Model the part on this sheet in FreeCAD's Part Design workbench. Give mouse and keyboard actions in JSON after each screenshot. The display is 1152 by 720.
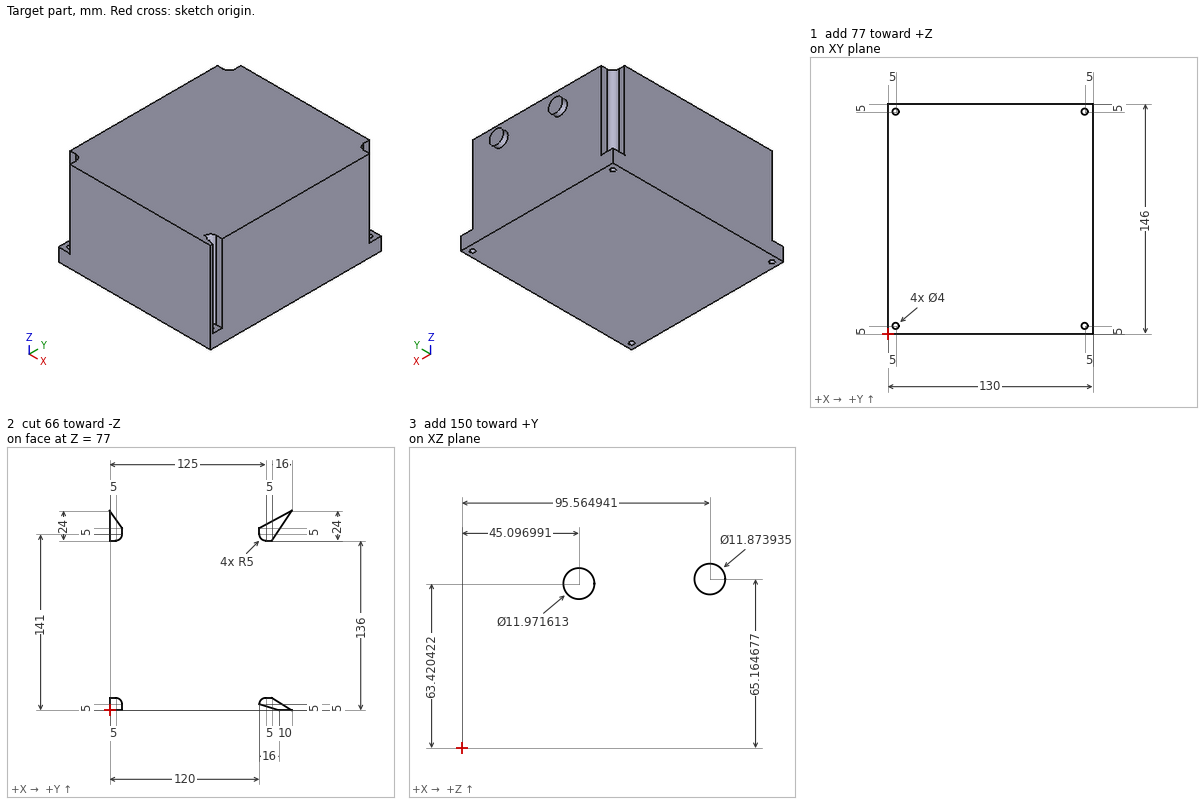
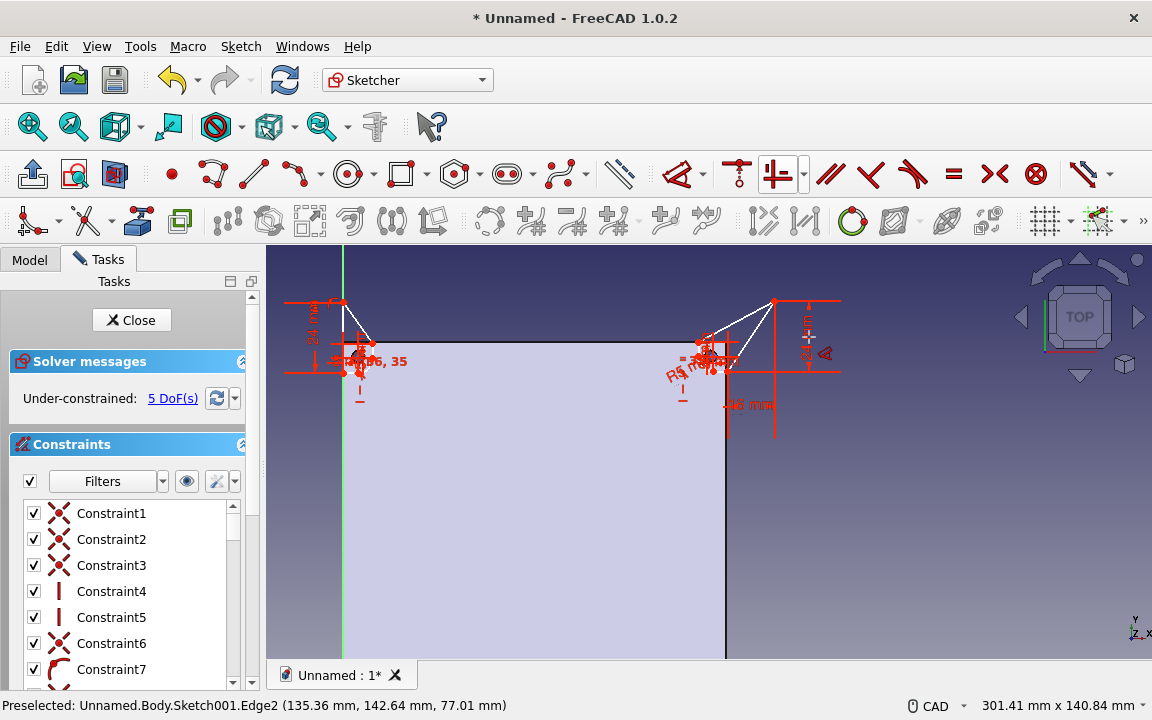
{"action": "scroll", "coordinate": [741, 350], "scroll_direction": "down", "scroll_amount": 3}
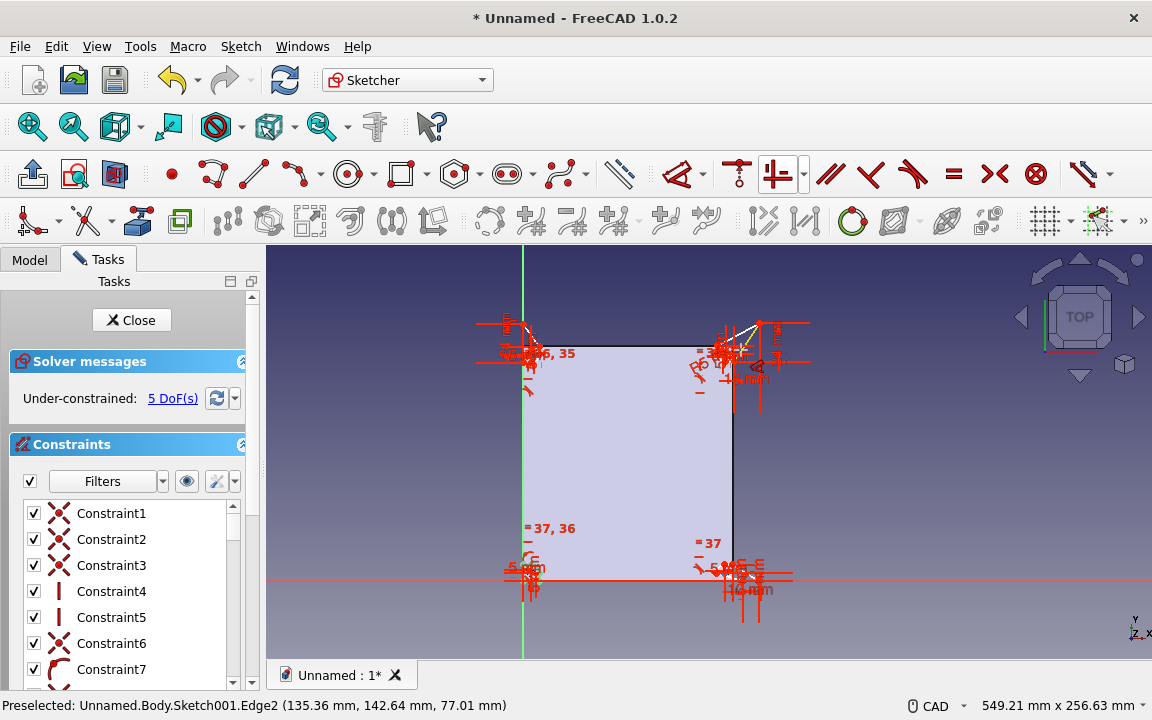
{"action": "scroll", "coordinate": [724, 575], "scroll_direction": "up", "scroll_amount": 5}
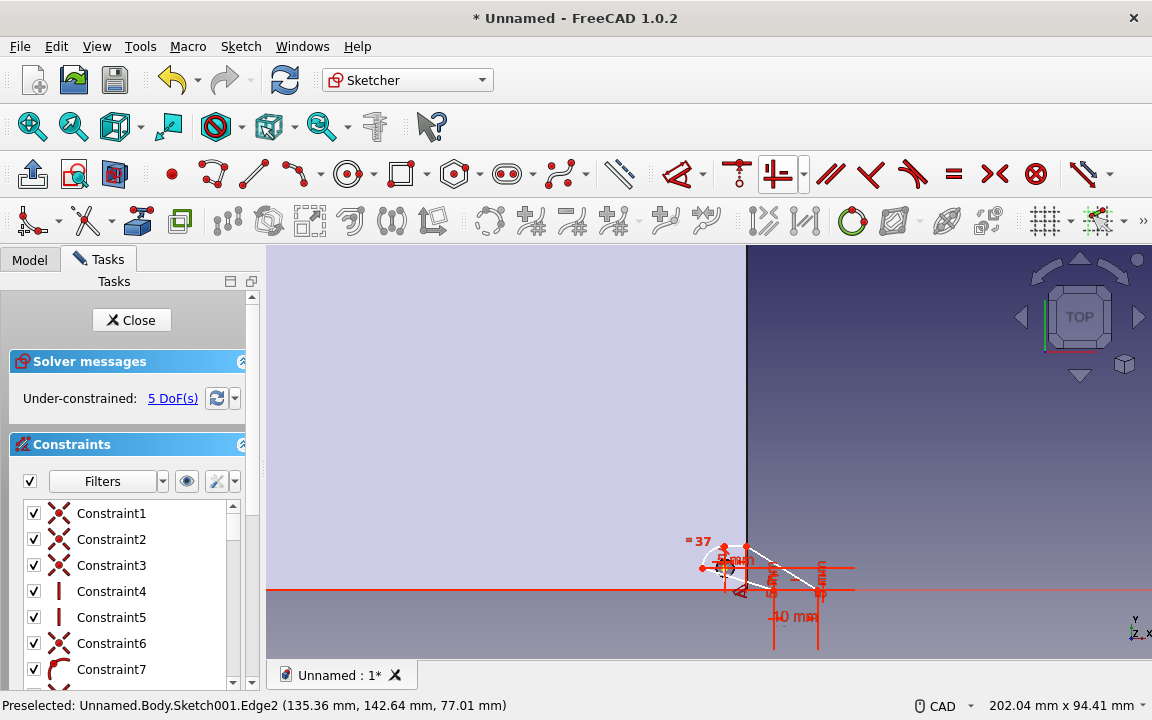
{"action": "left_click", "coordinate": [724, 575]}
{"action": "left_click", "coordinate": [722, 624]}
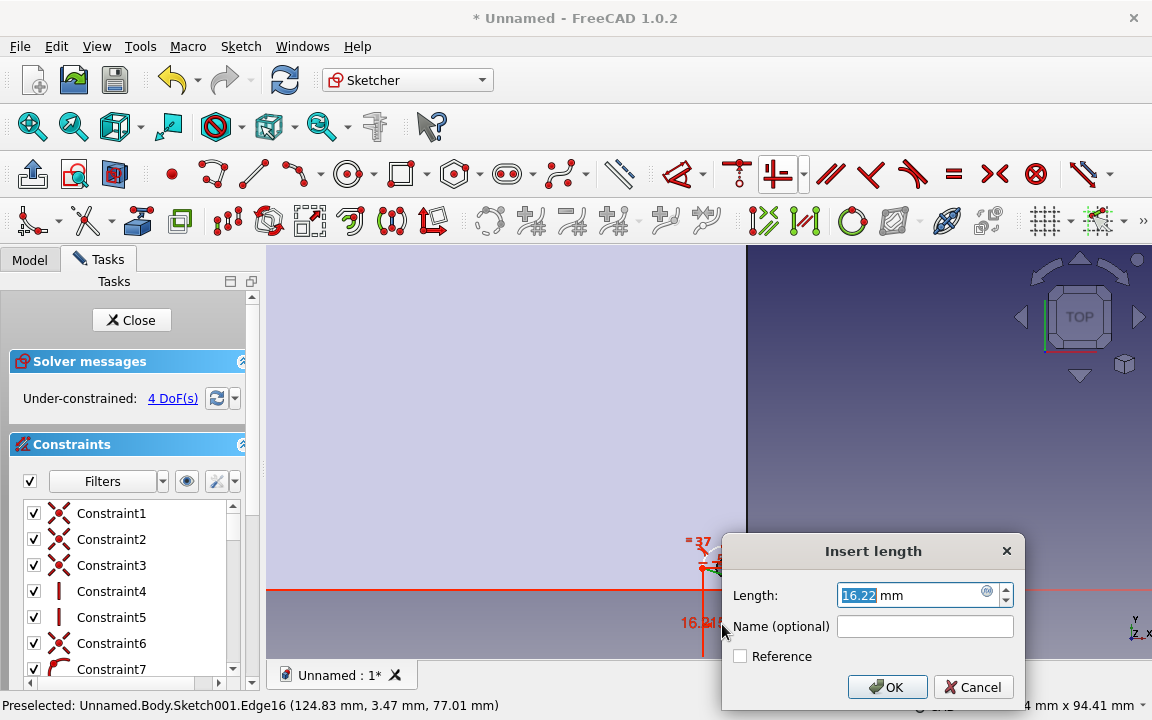
{"action": "type", "text": "16"}
{"action": "key", "text": "Return"}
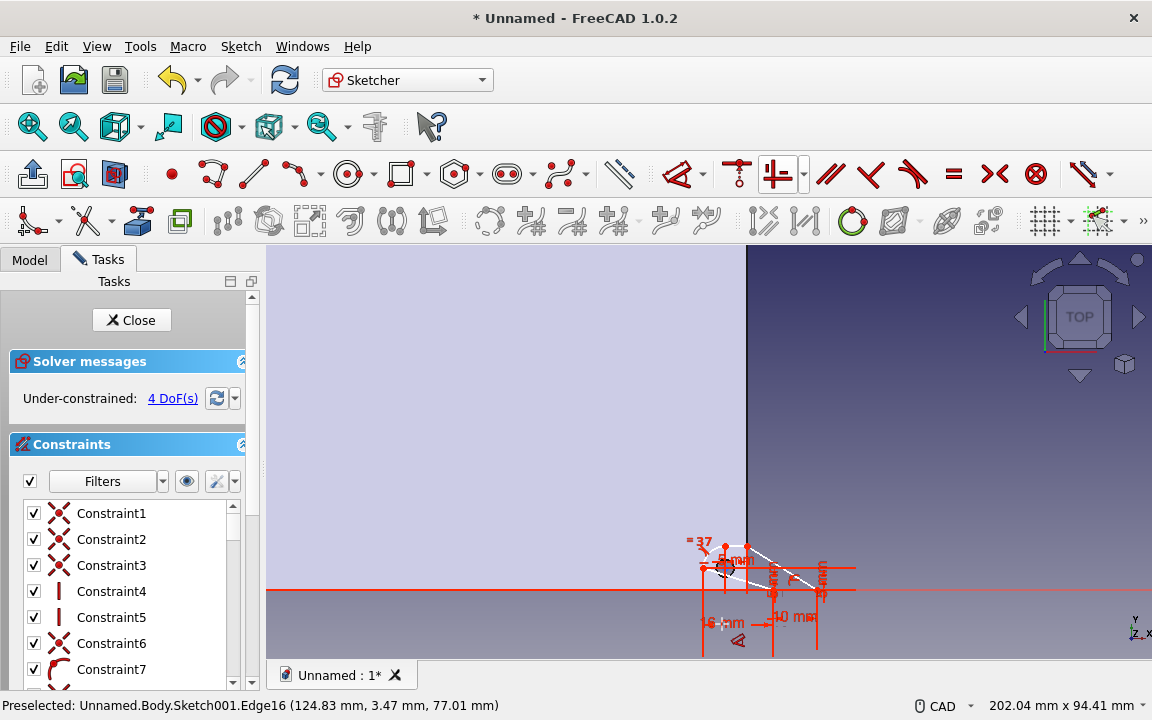
{"action": "scroll", "coordinate": [724, 576], "scroll_direction": "down", "scroll_amount": 5}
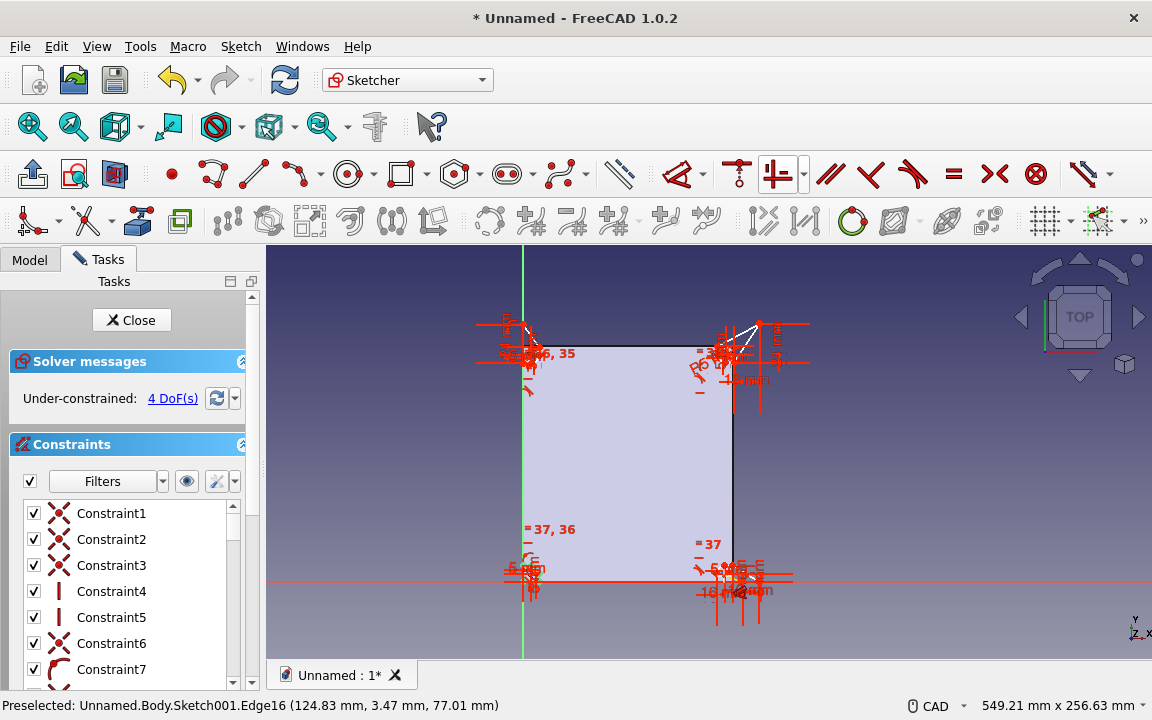
{"action": "scroll", "coordinate": [726, 363], "scroll_direction": "up", "scroll_amount": 3}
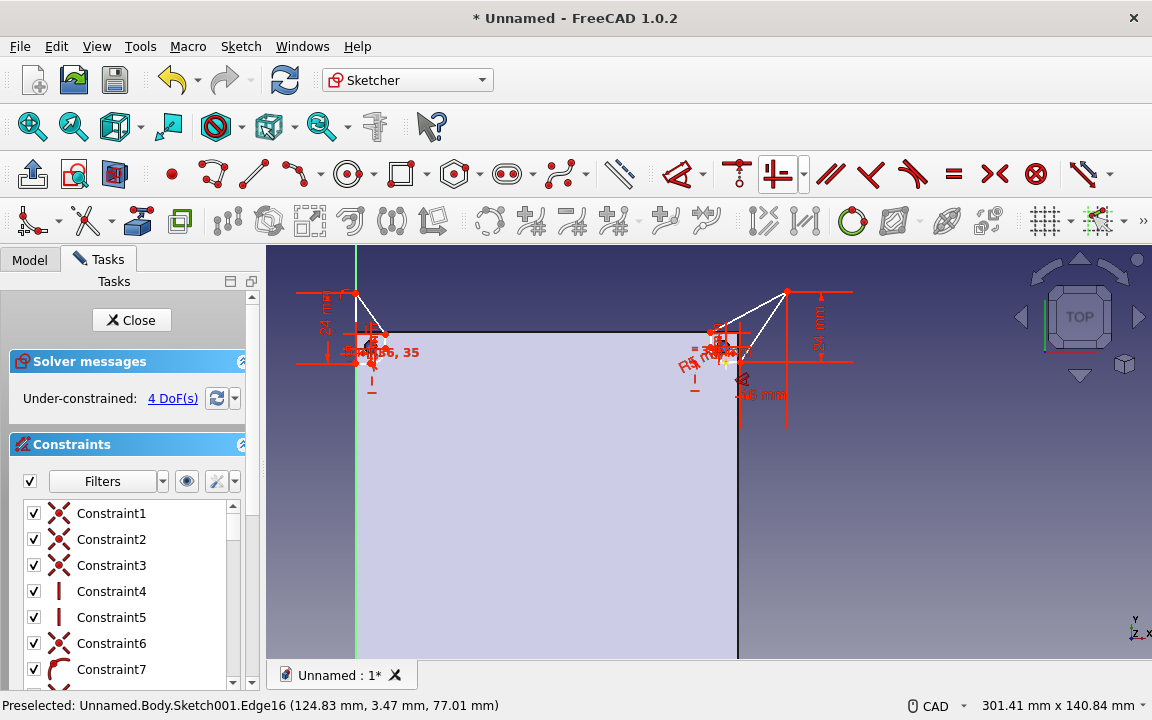
{"action": "left_click", "coordinate": [726, 362]}
{"action": "left_click", "coordinate": [541, 328]}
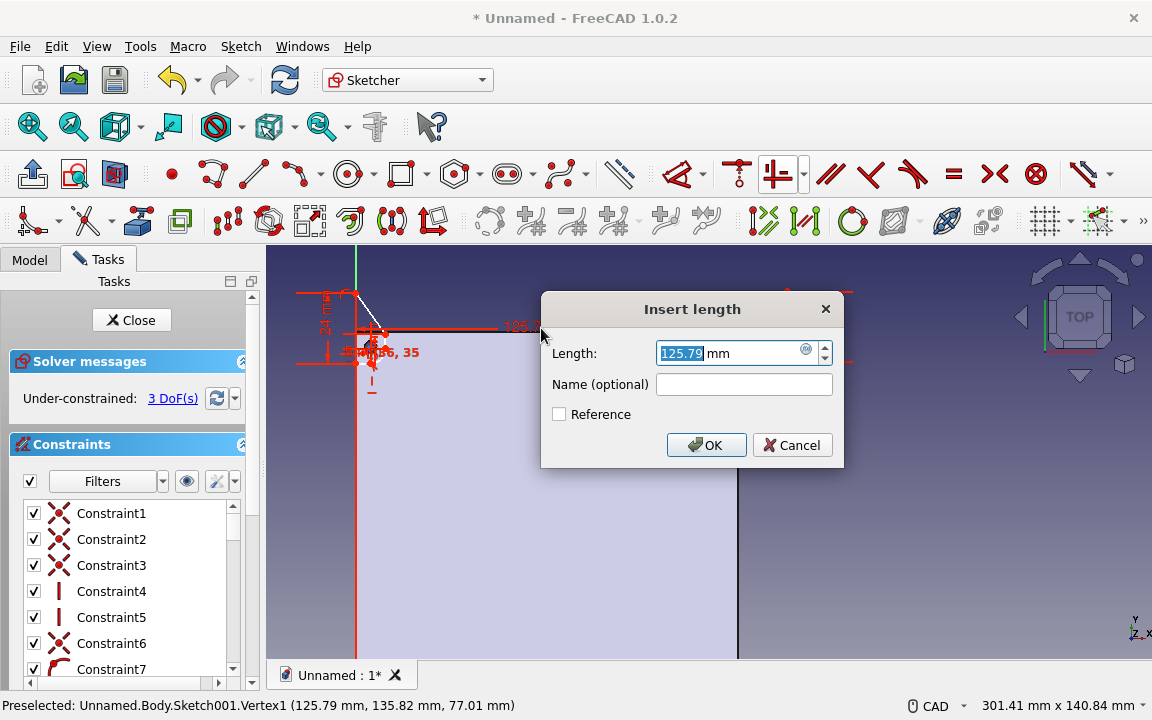
{"action": "type", "text": "125"}
{"action": "key", "text": "Return"}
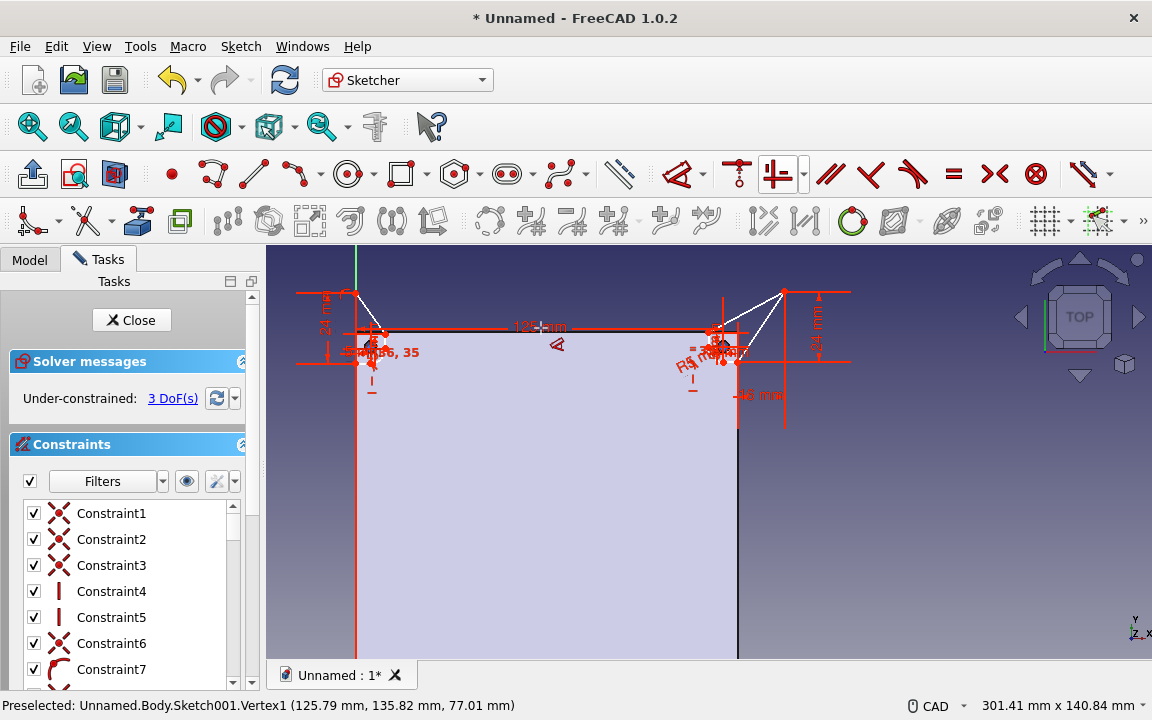
{"action": "left_click", "coordinate": [723, 362]}
{"action": "left_click", "coordinate": [322, 497]}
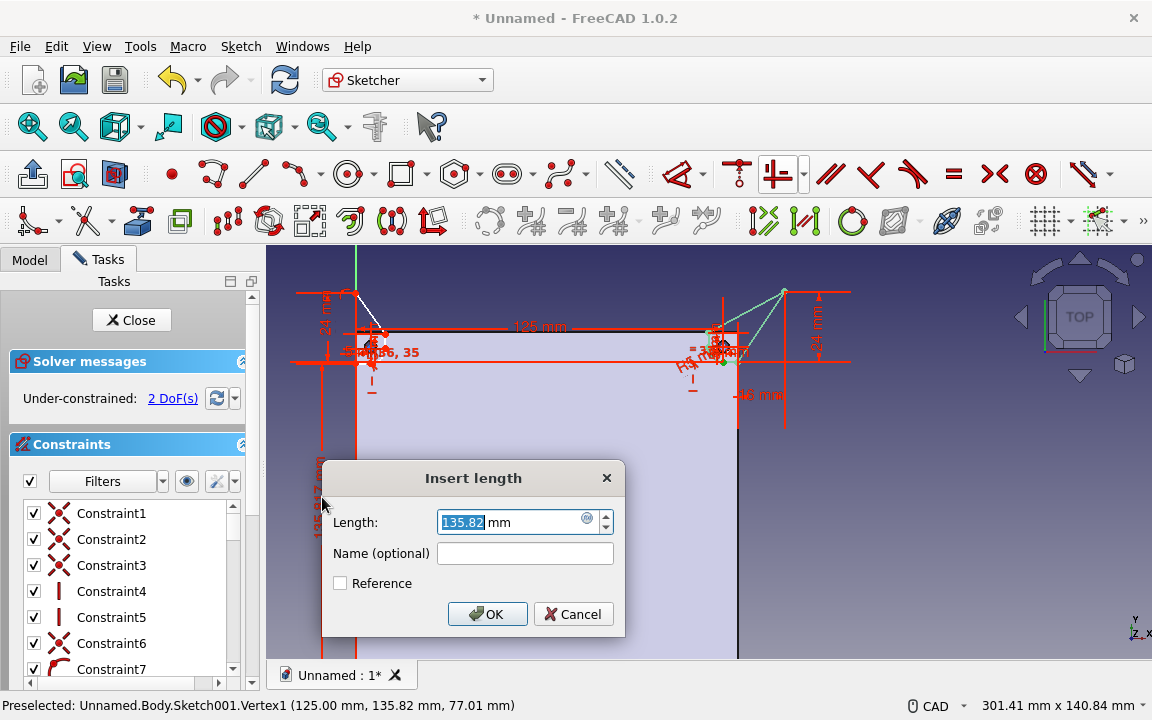
{"action": "type", "text": "136"}
{"action": "key", "text": "Return"}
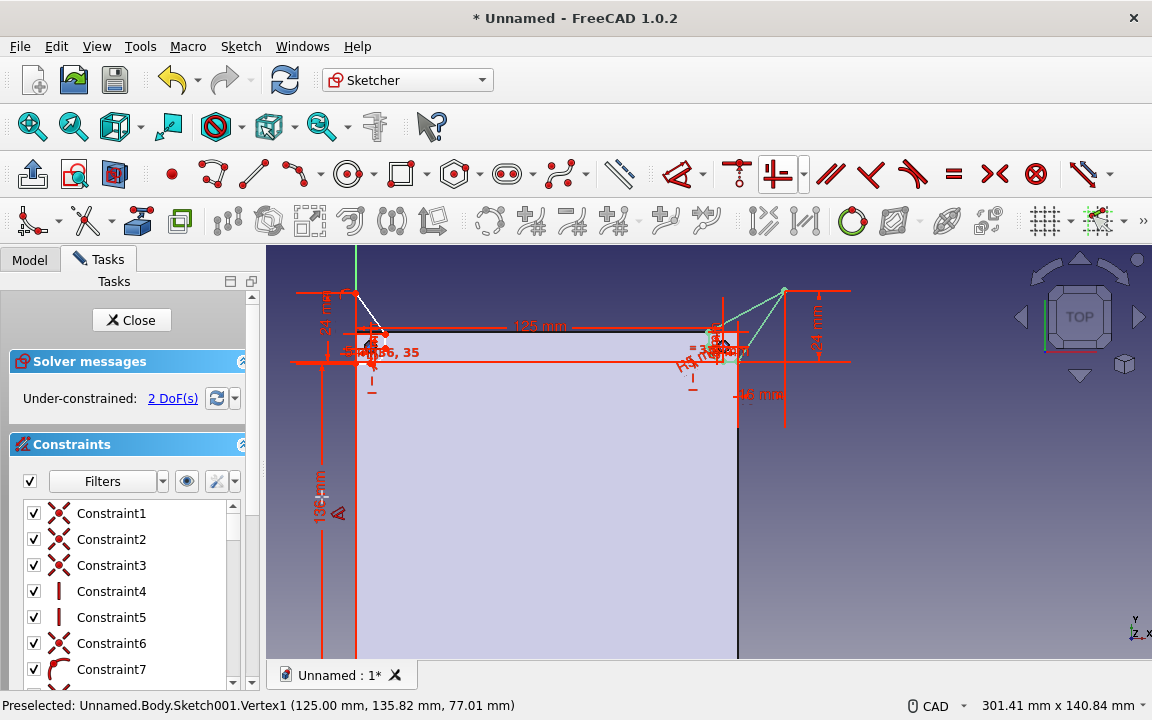
{"action": "left_click", "coordinate": [385, 349]}
{"action": "left_click", "coordinate": [322, 425]}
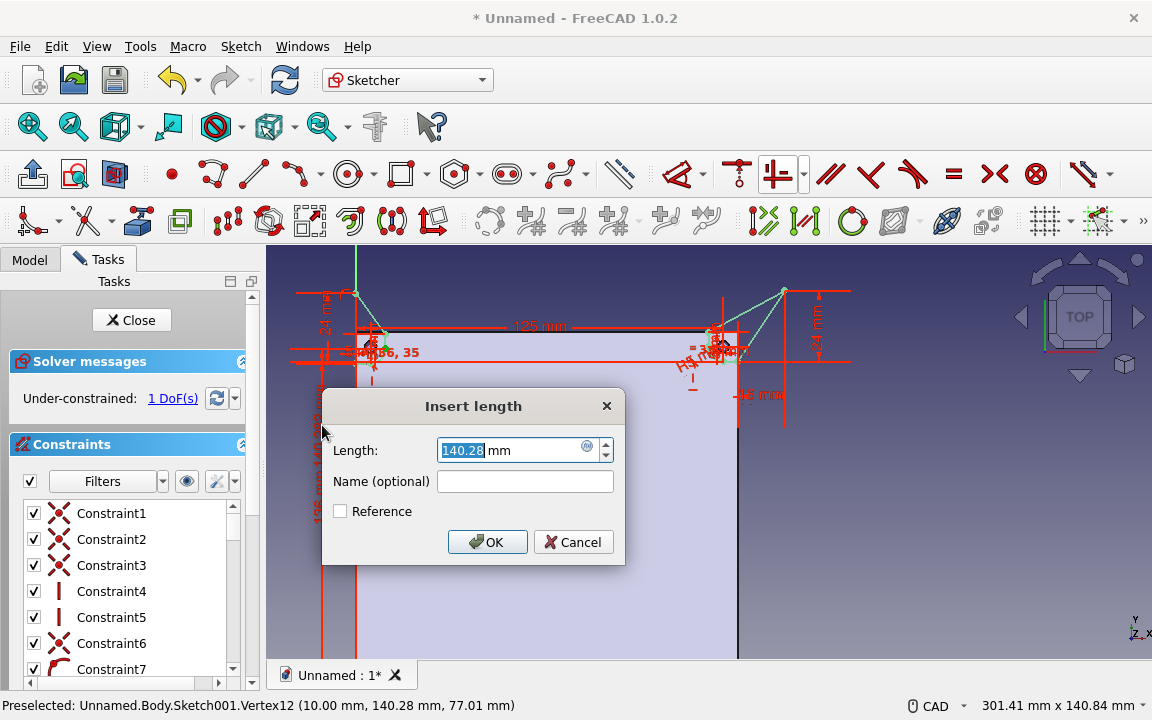
{"action": "type", "text": "141"}
{"action": "key", "text": "Return"}